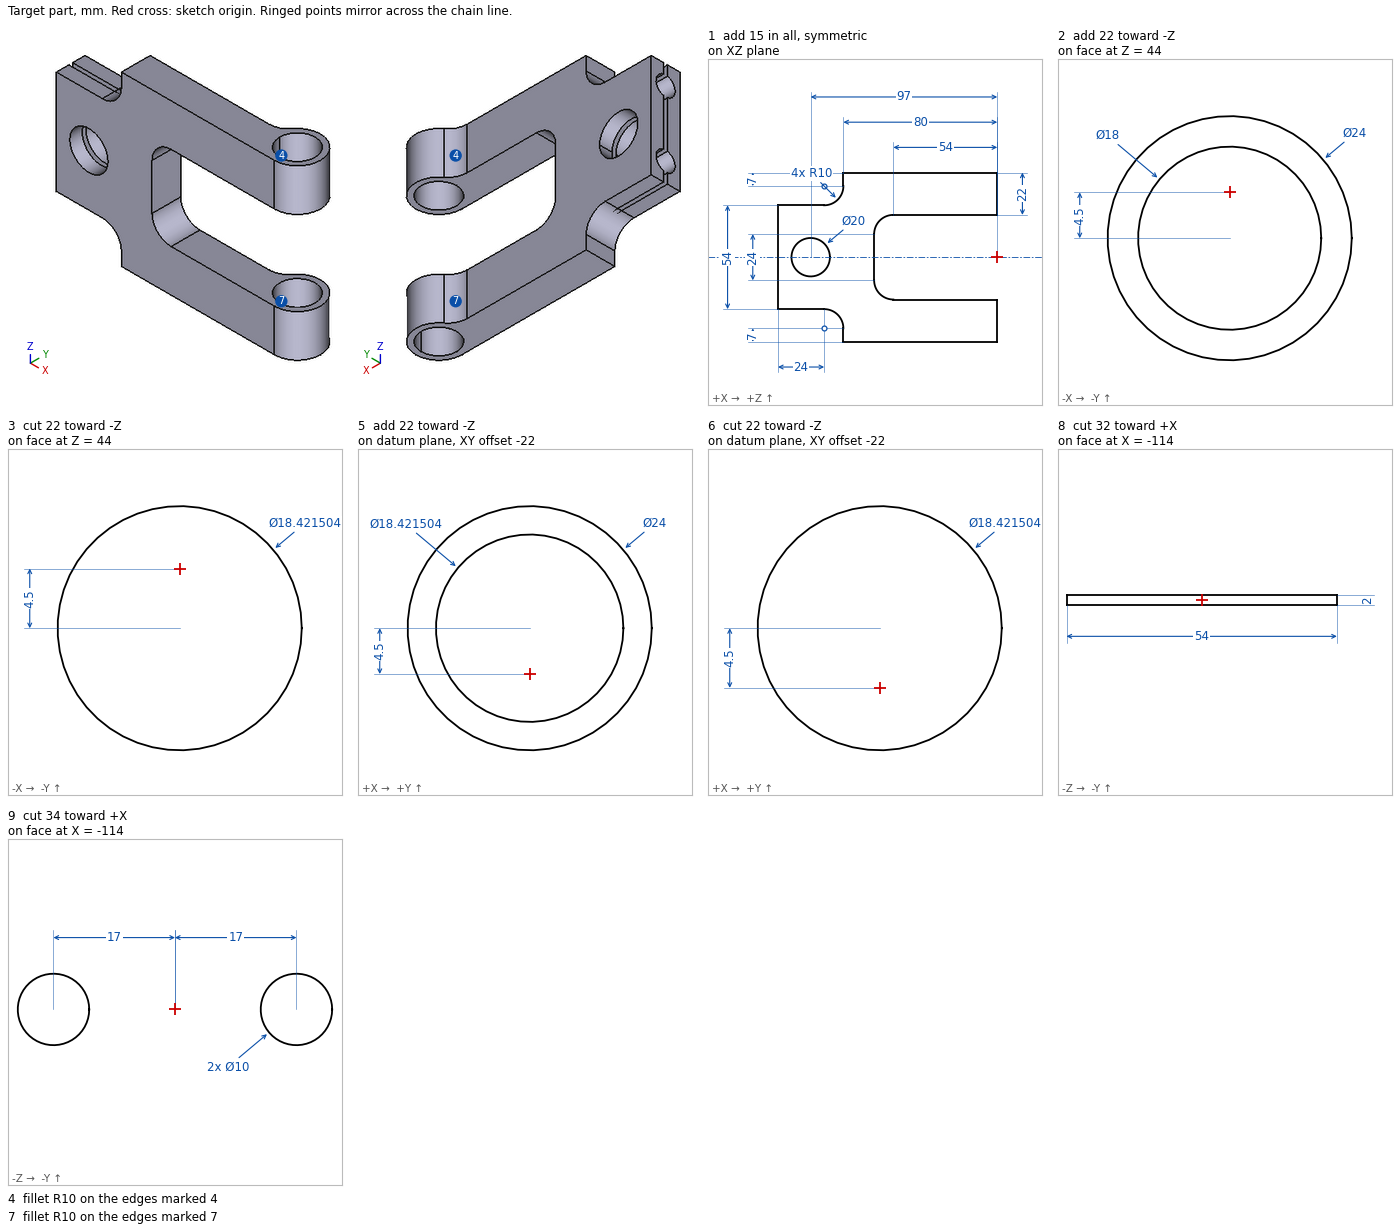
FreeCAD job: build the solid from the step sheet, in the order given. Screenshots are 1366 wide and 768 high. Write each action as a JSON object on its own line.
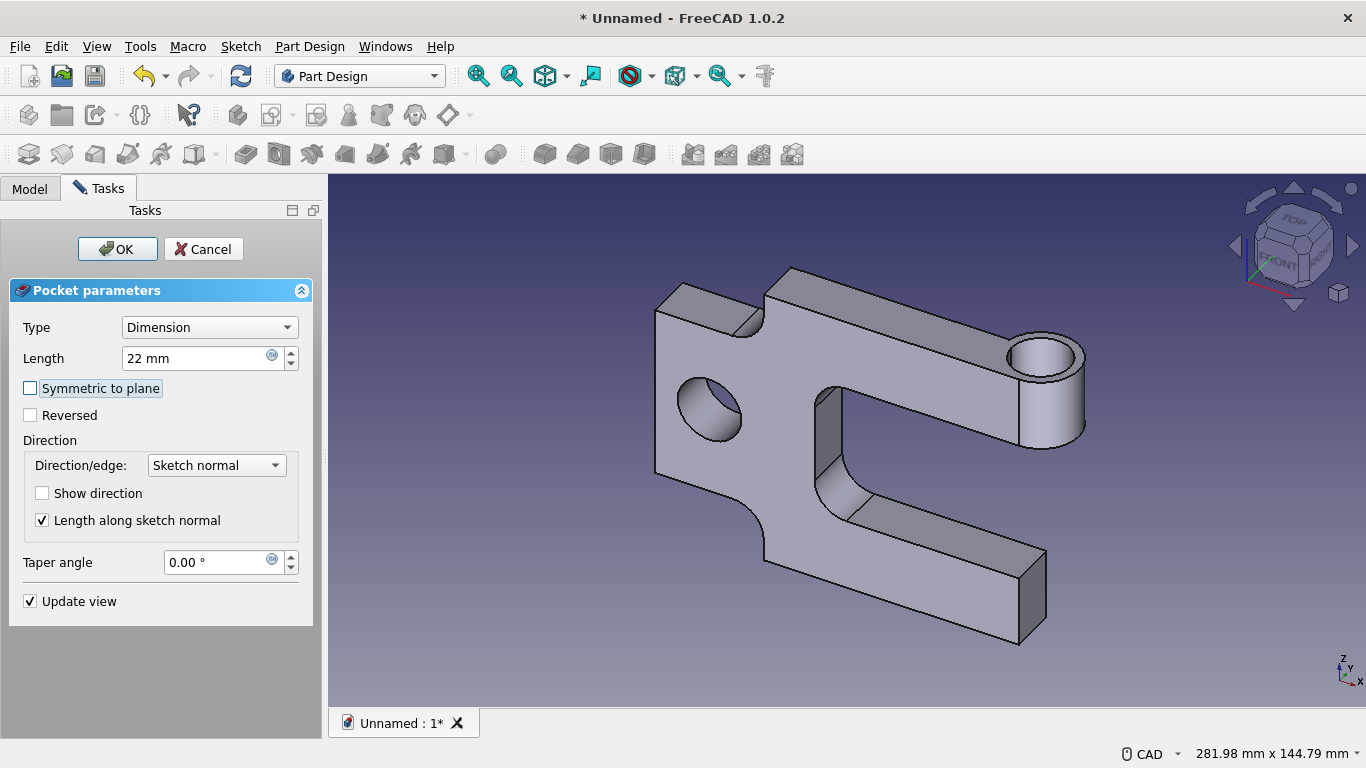
{"action": "left_click", "coordinate": [118, 249]}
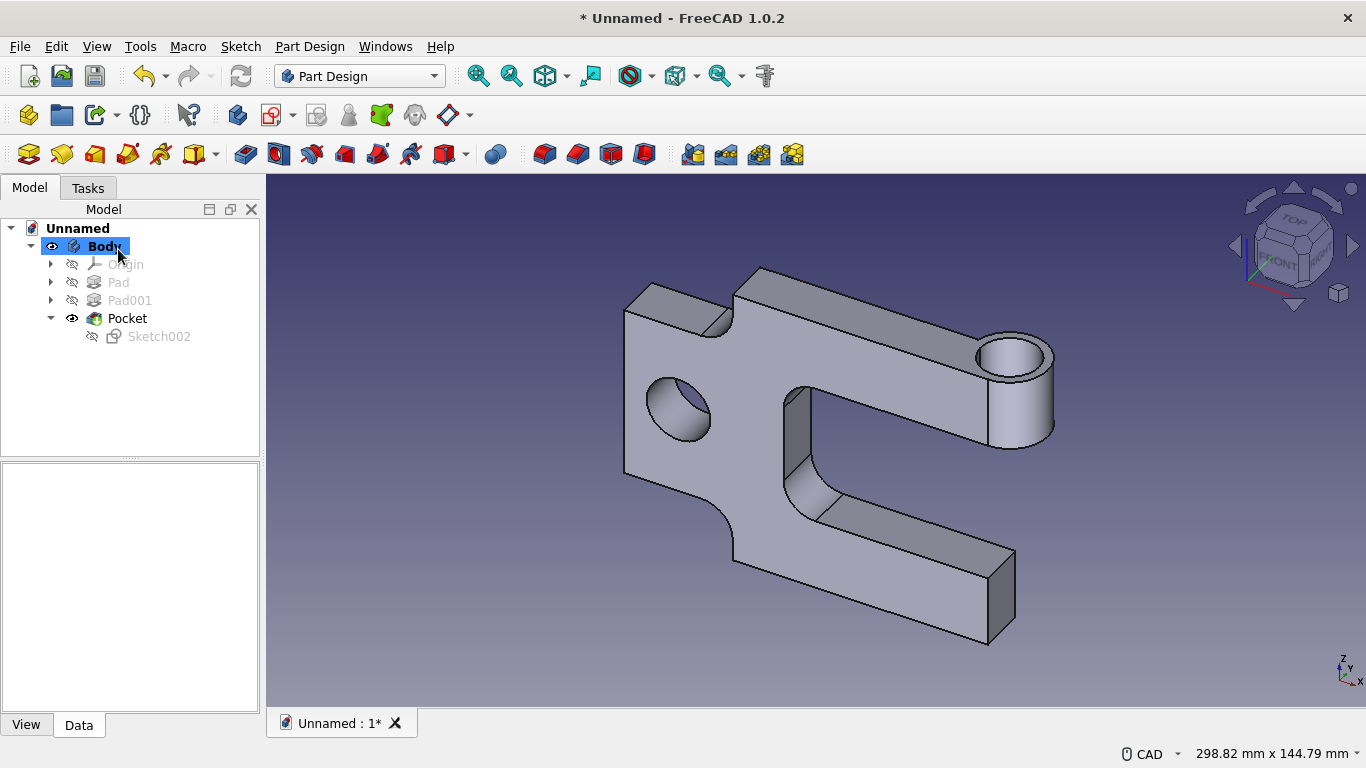
{"action": "key", "text": "0"}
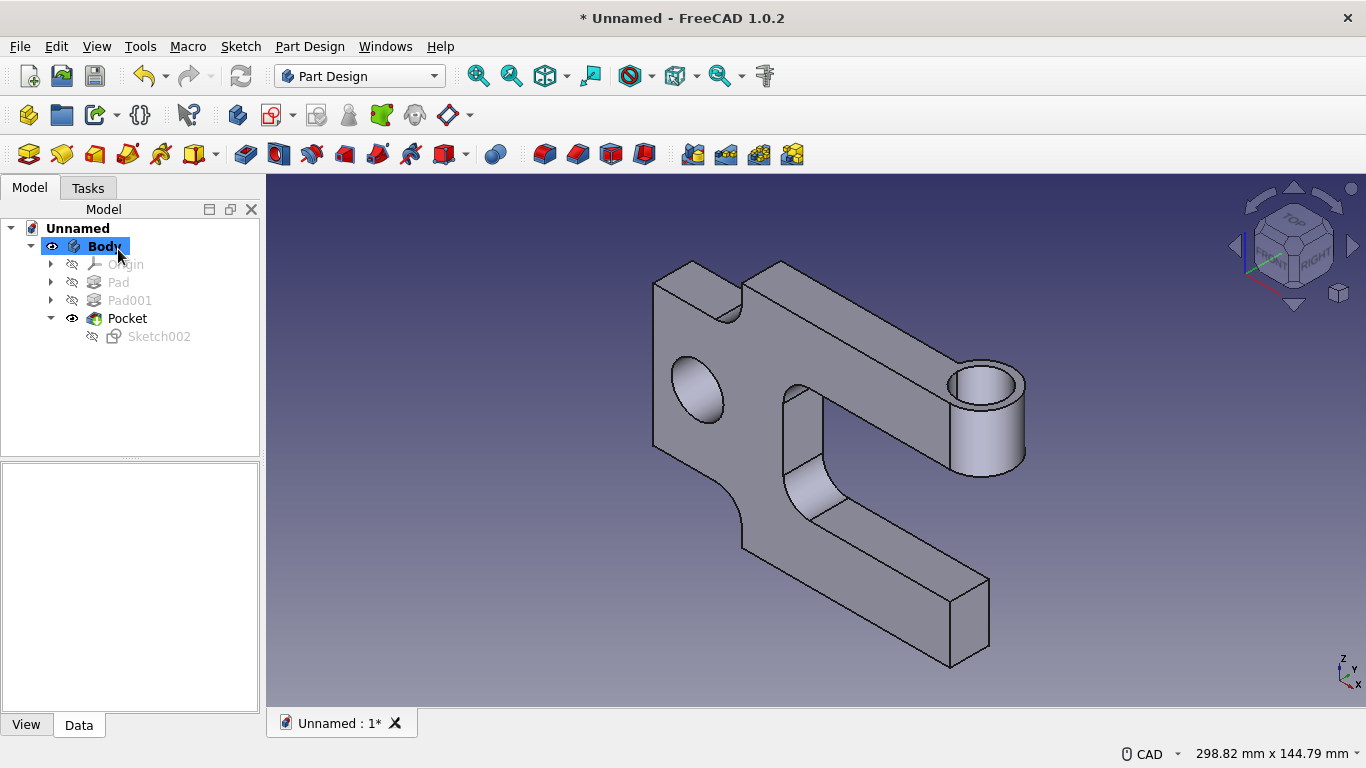
{"action": "key", "text": "2"}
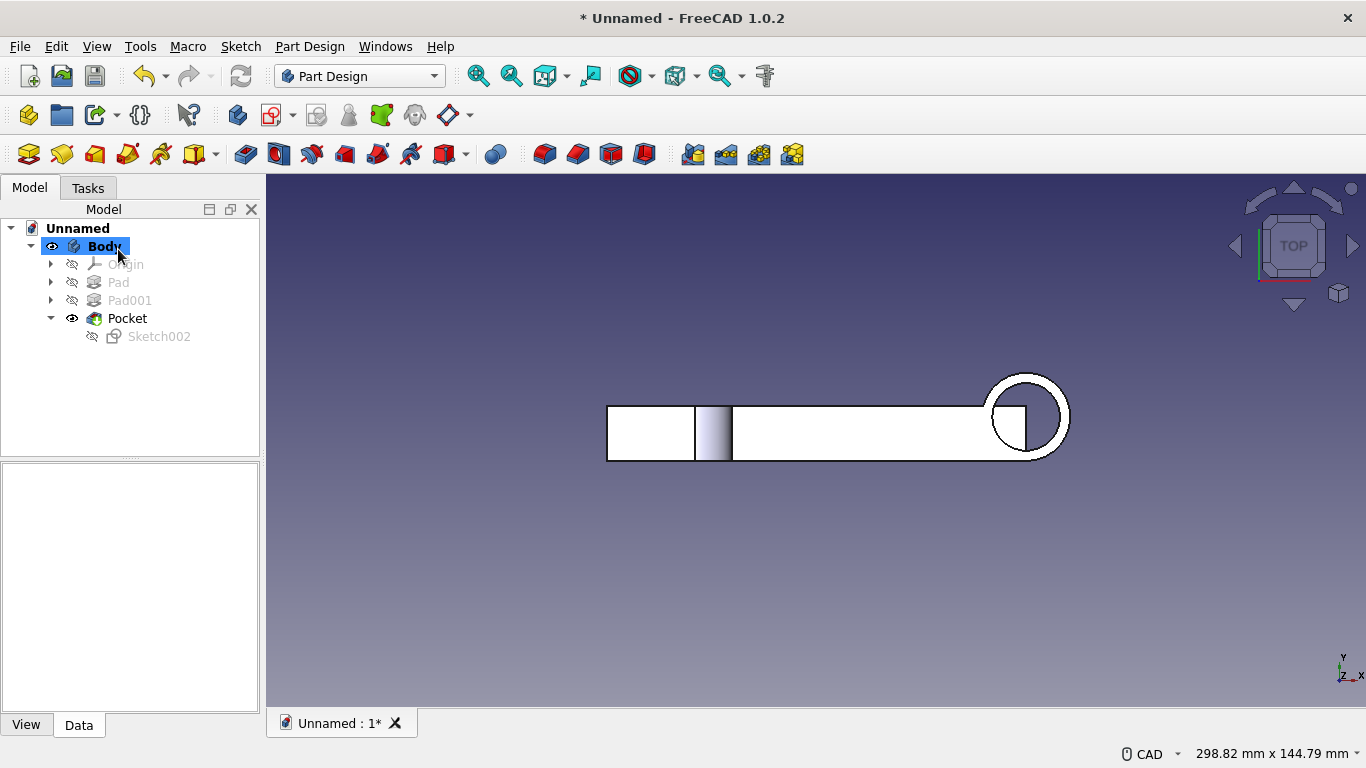
{"action": "left_click", "coordinate": [479, 76]}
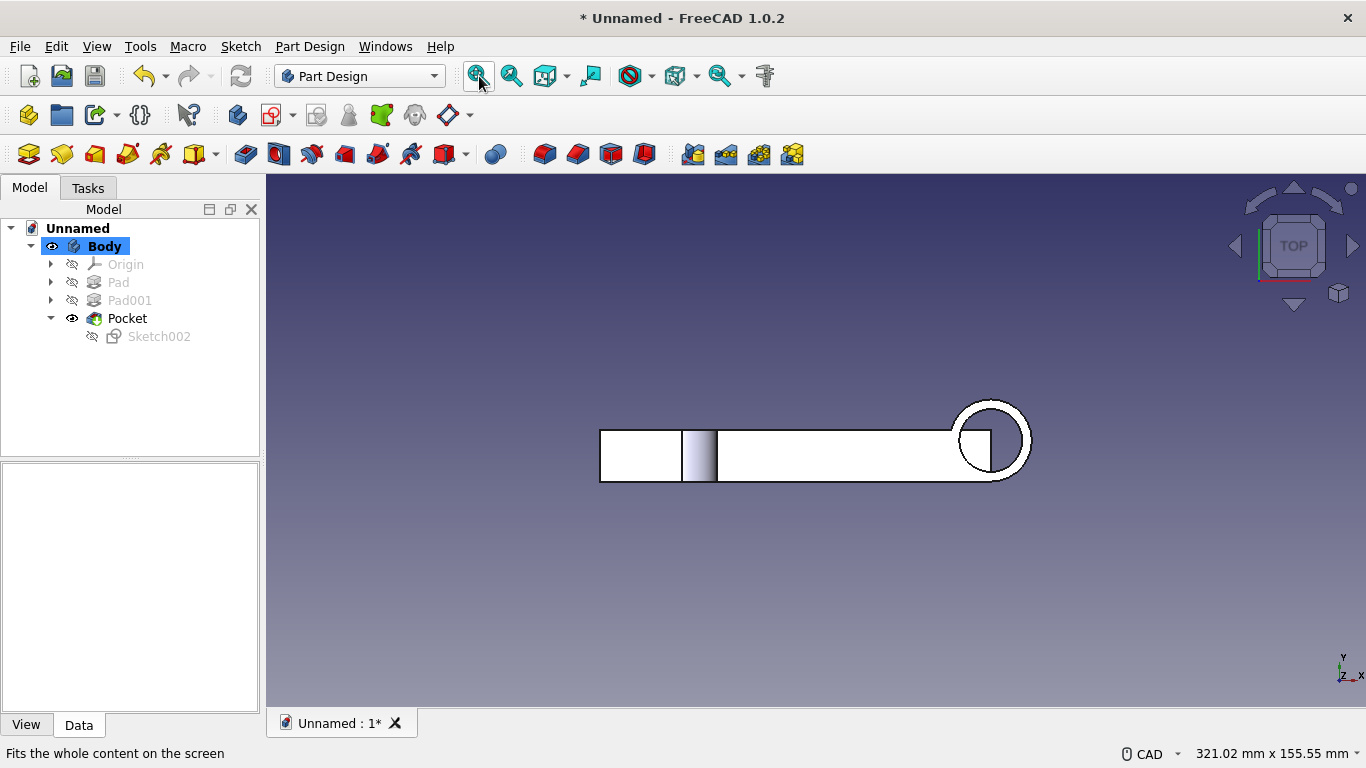
{"action": "key", "text": "1"}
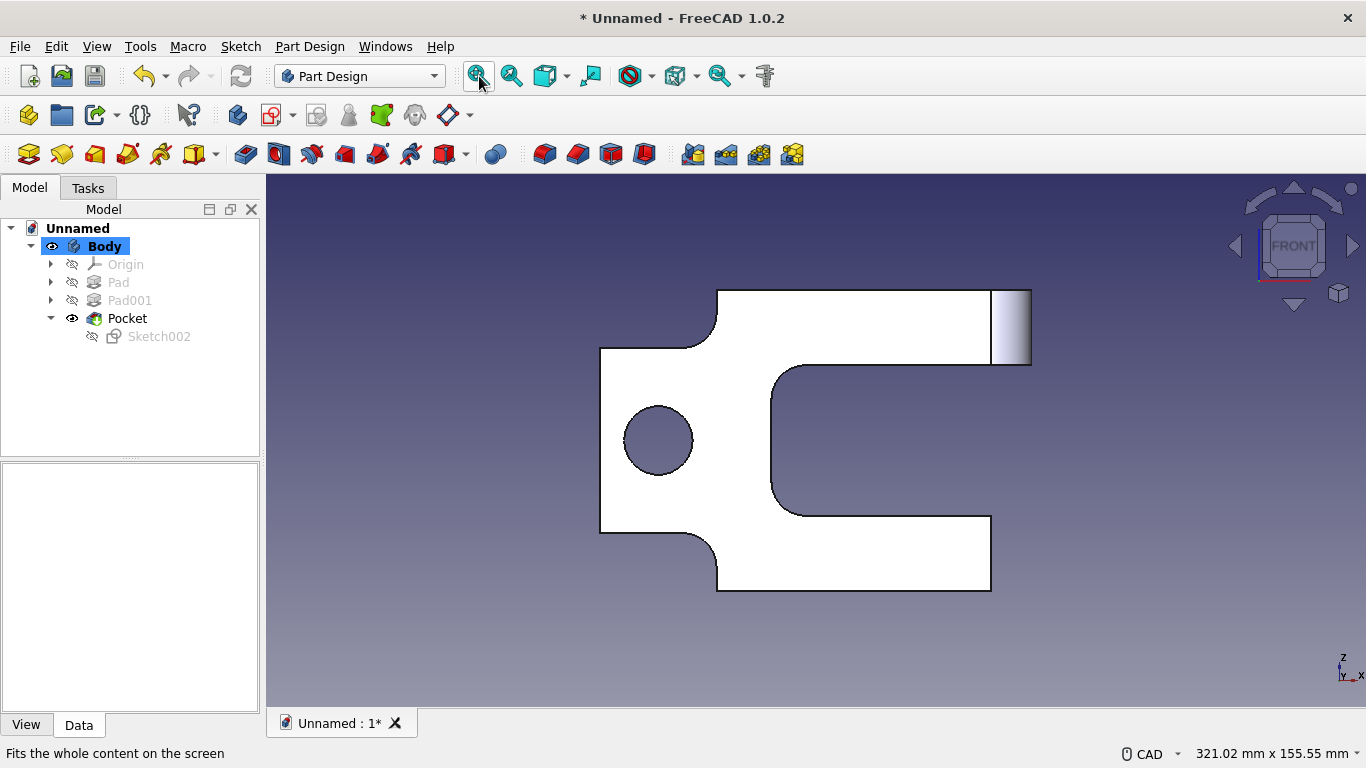
{"action": "key", "text": "3"}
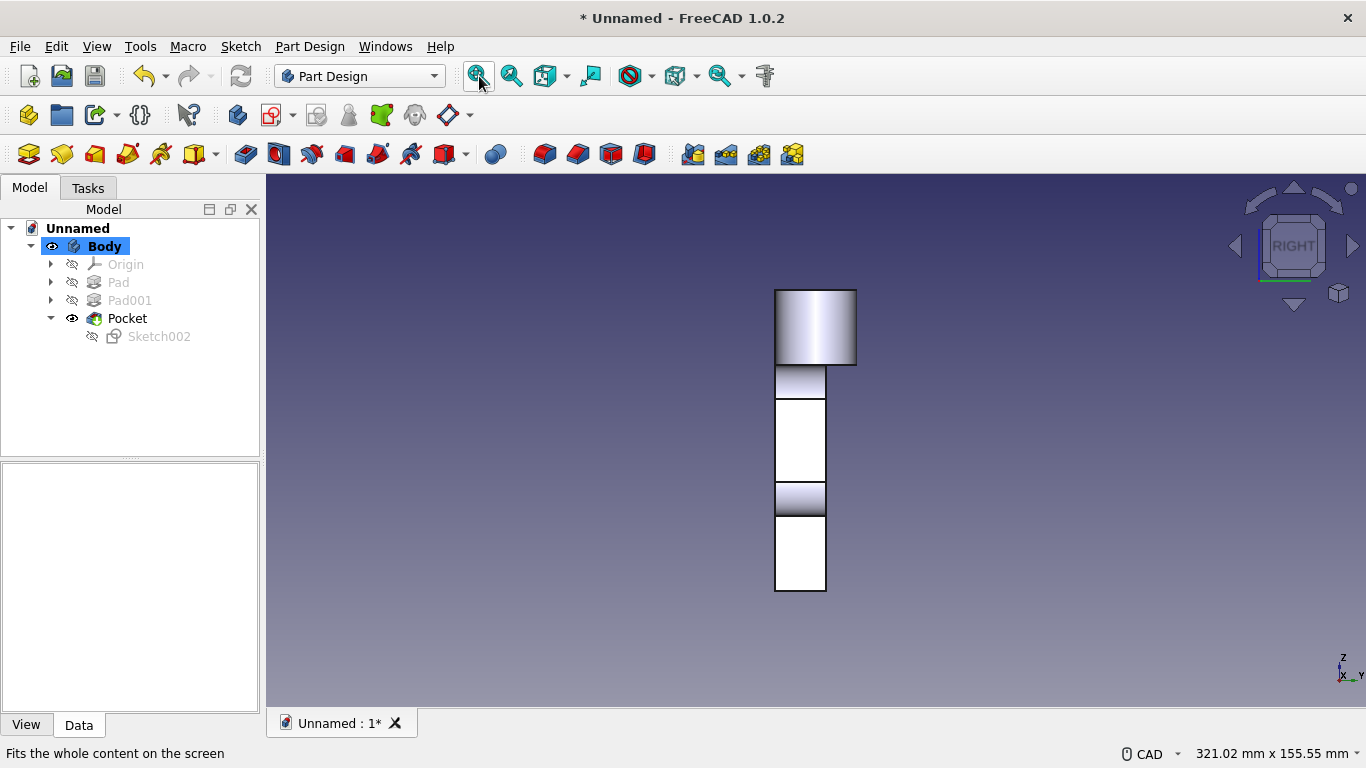
{"action": "key", "text": "5"}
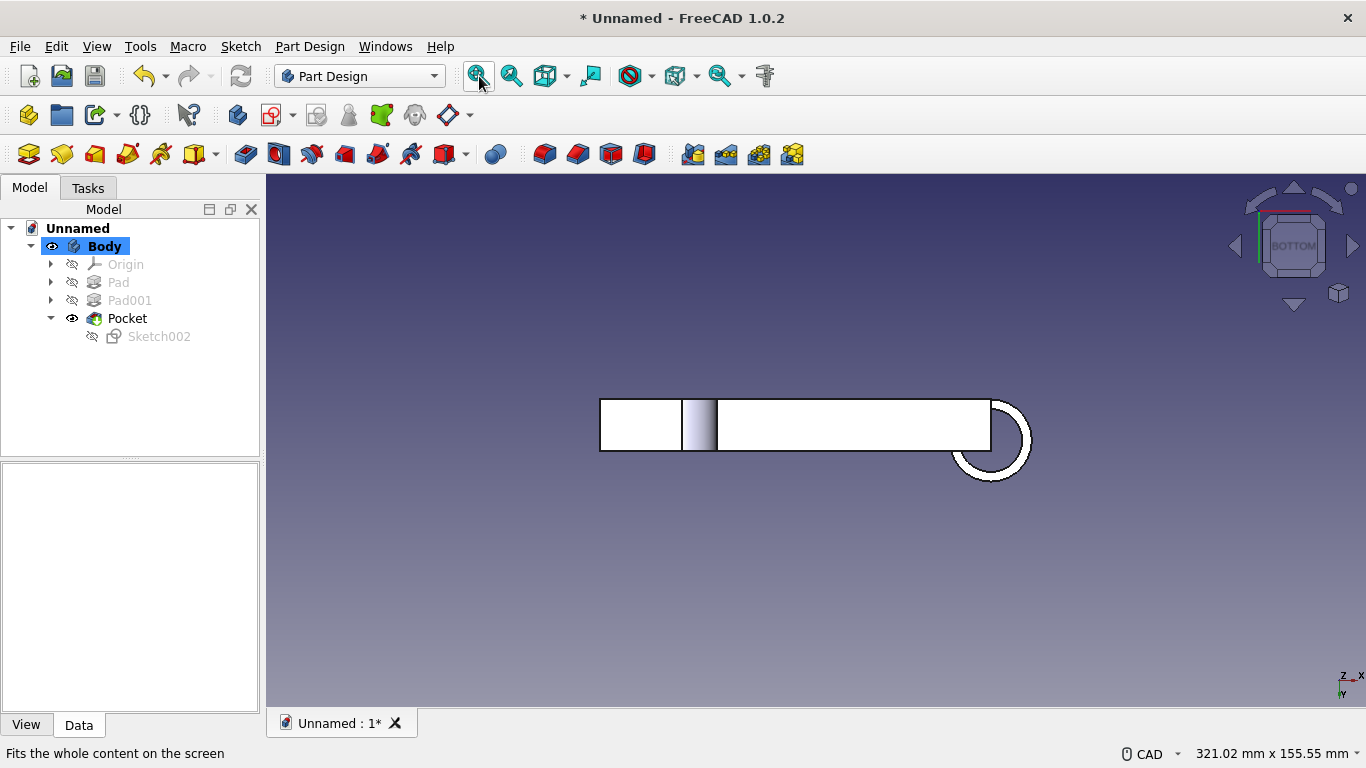
{"action": "left_click", "coordinate": [479, 76]}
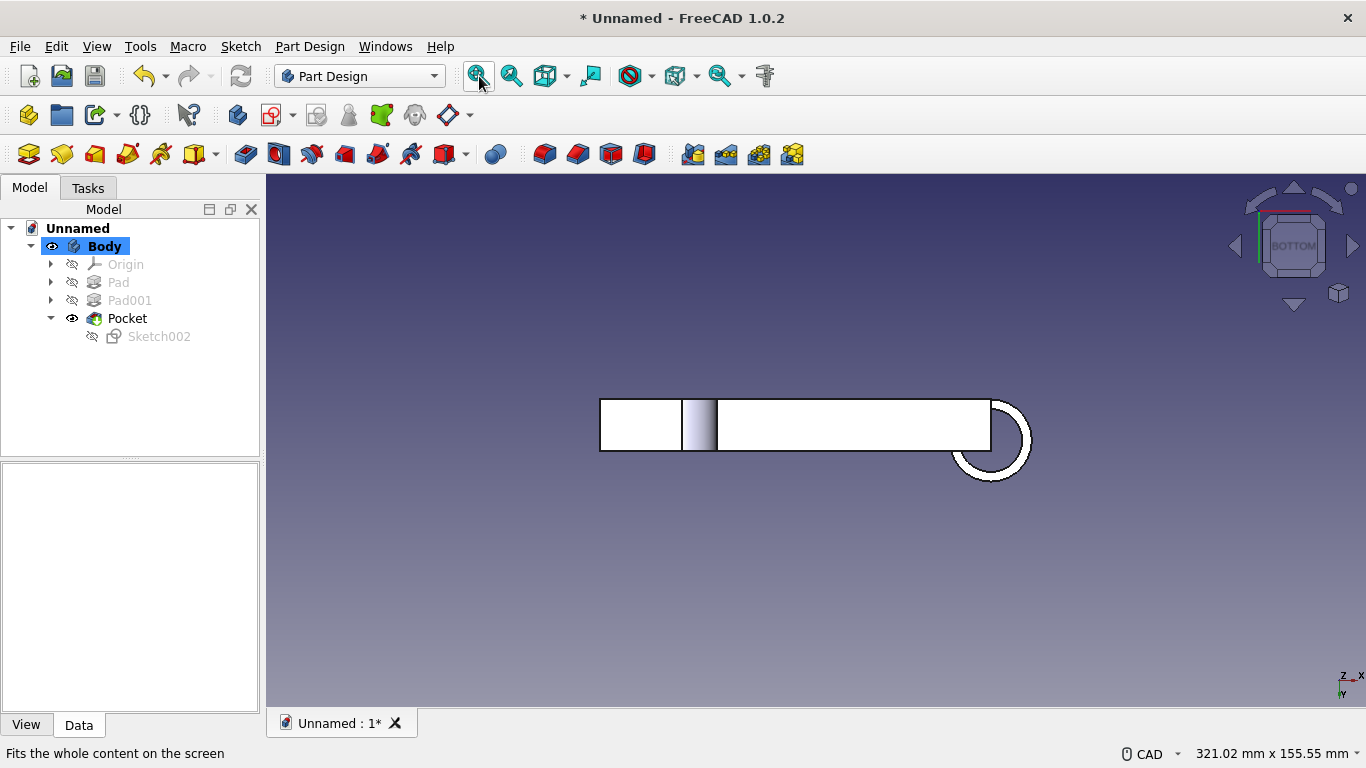
{"action": "key", "text": "4"}